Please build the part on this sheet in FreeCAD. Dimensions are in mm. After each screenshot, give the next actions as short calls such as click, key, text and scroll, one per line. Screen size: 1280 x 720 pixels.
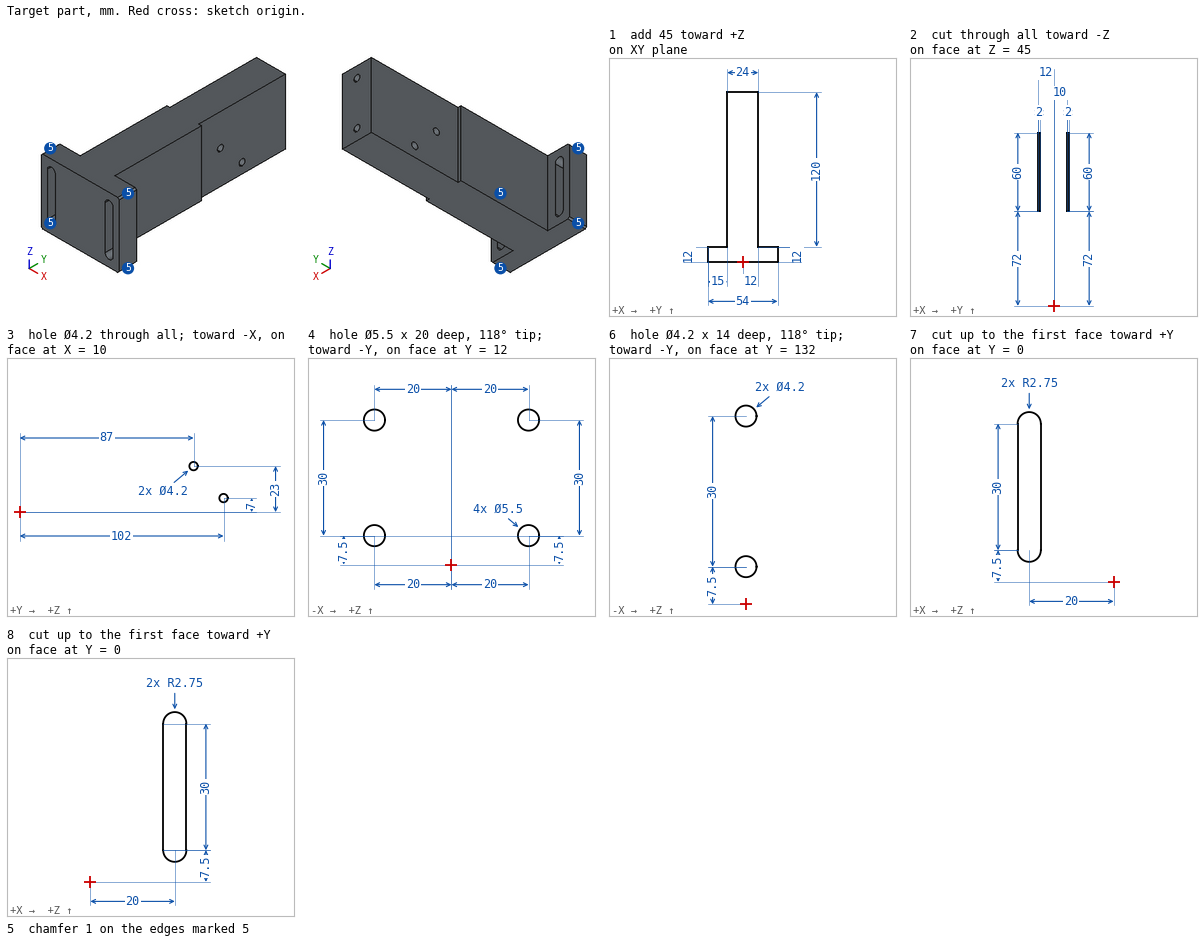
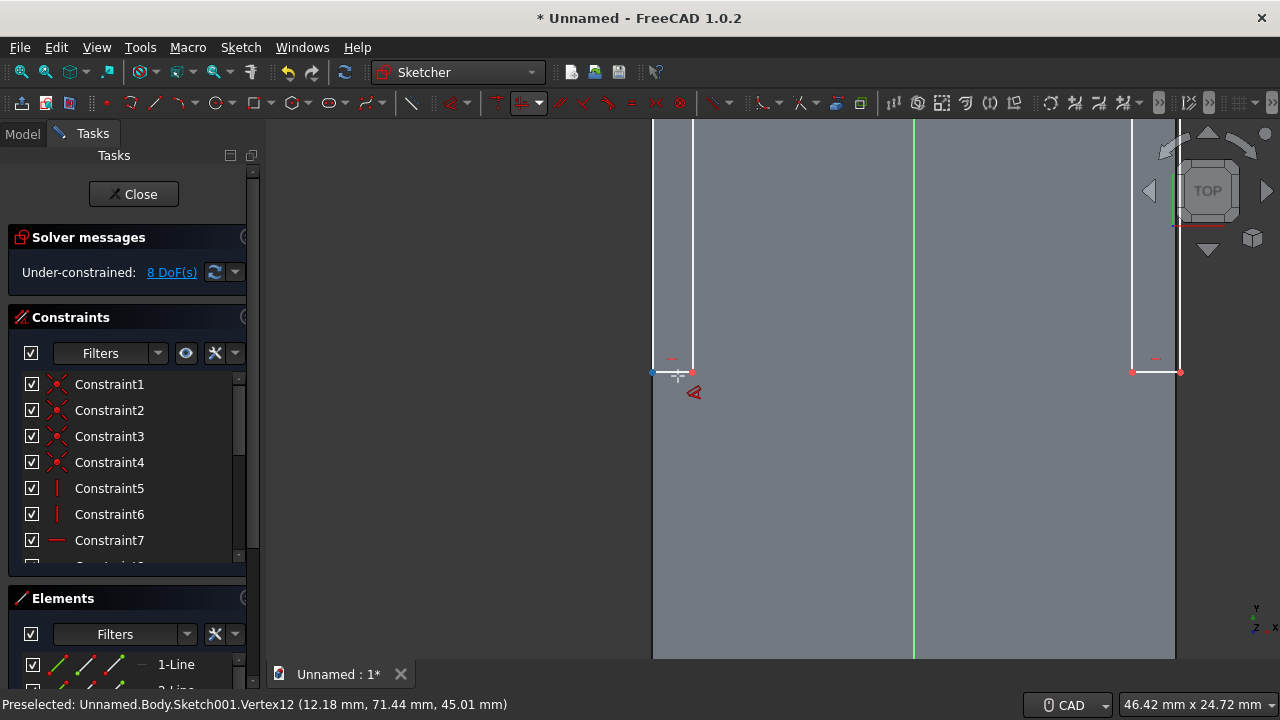
click(673, 372)
click(673, 338)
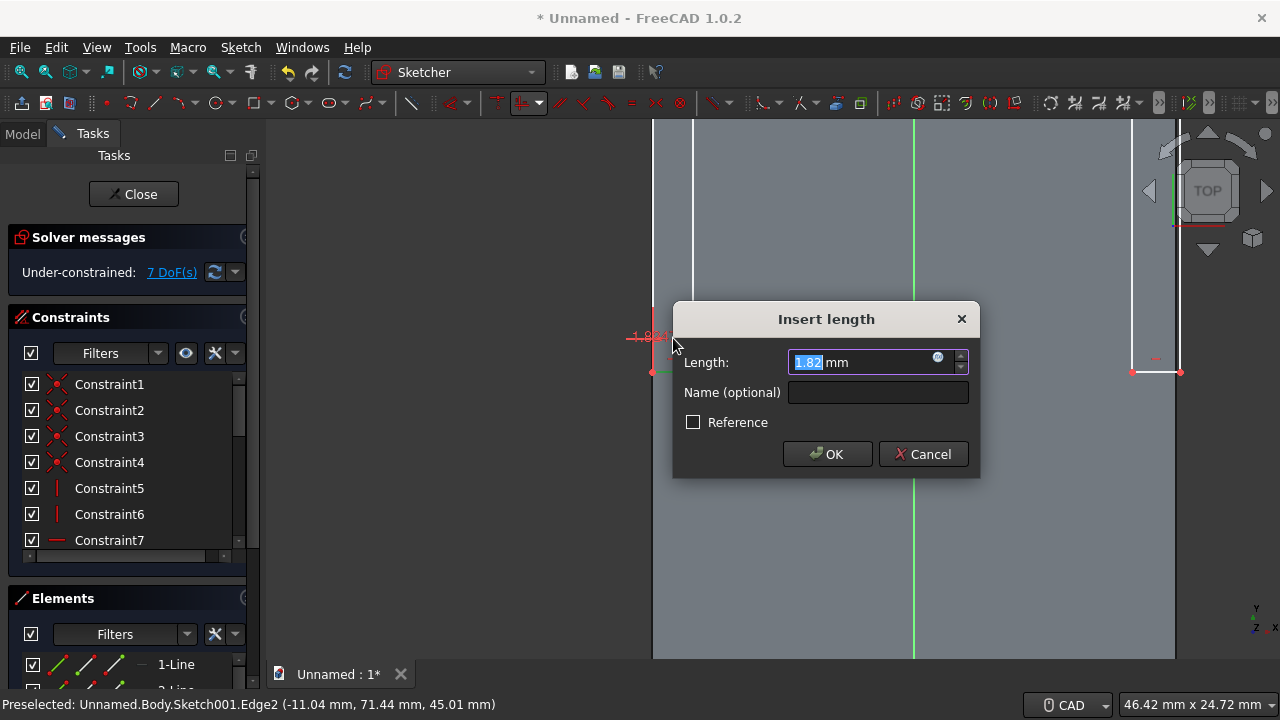
text(2)
key(Return)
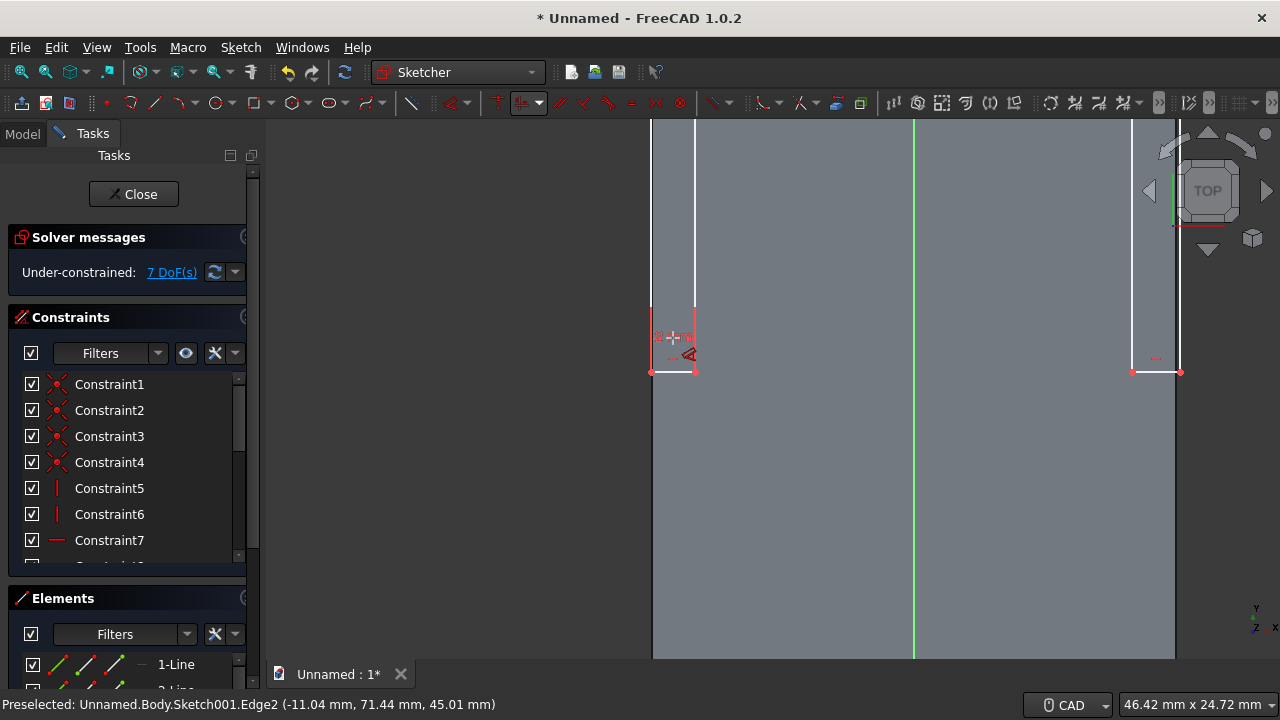
scroll(678, 376, down, 11)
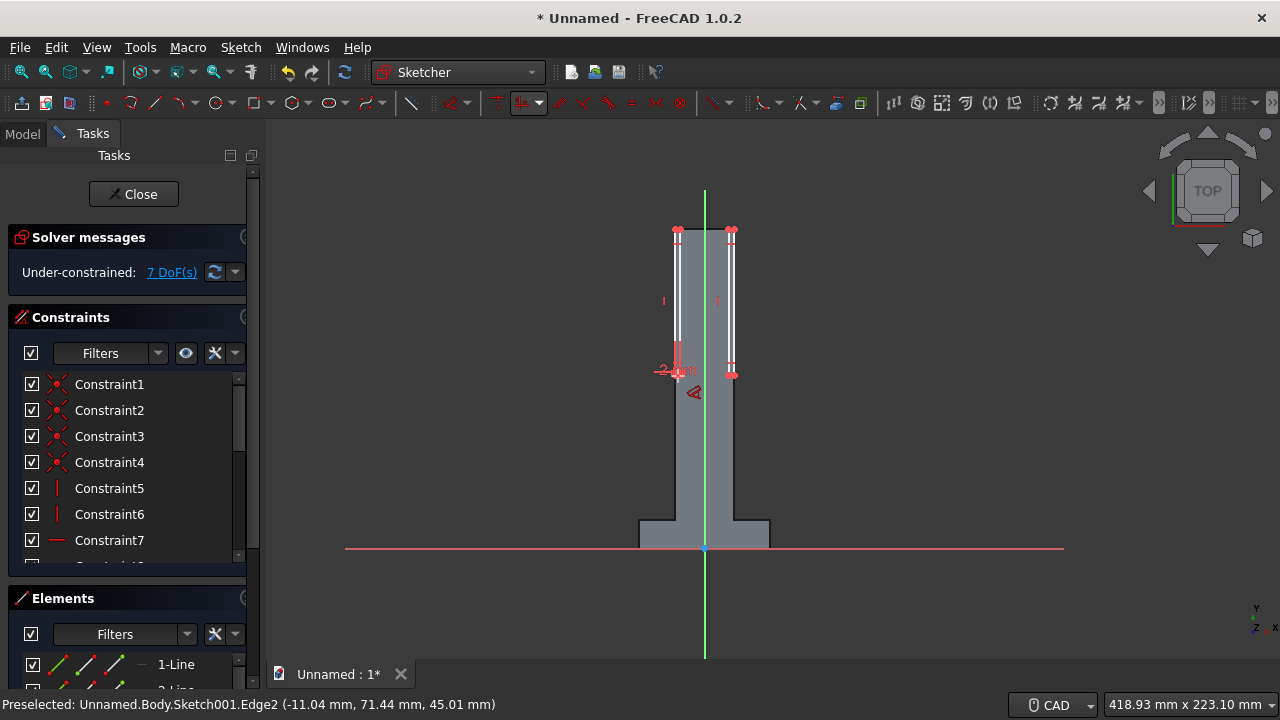
scroll(730, 376, up, 11)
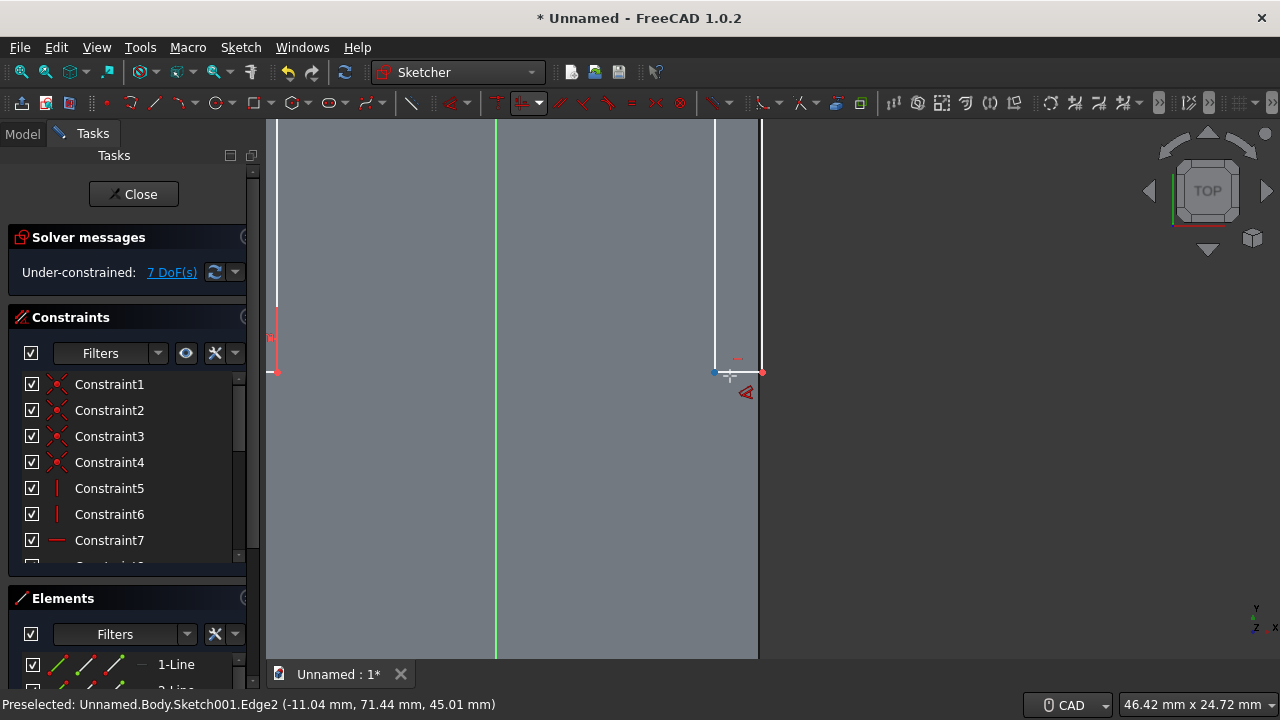
click(729, 372)
click(739, 338)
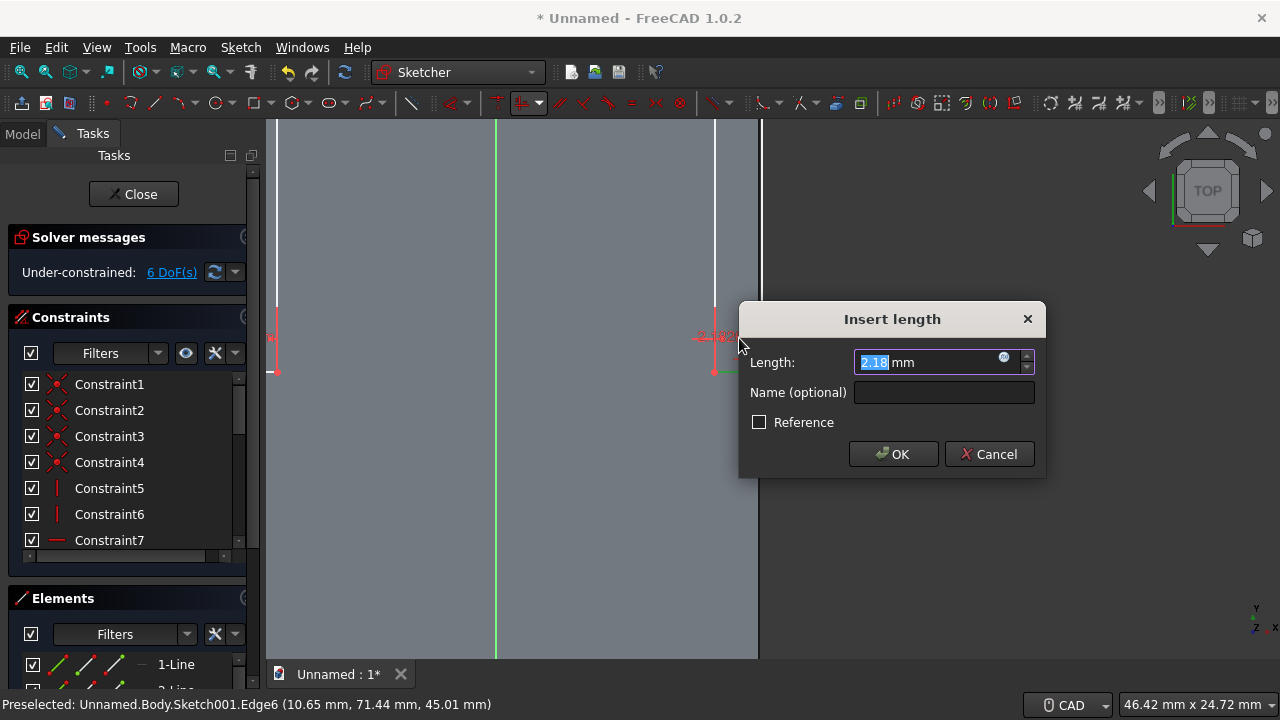
text(2)
key(Return)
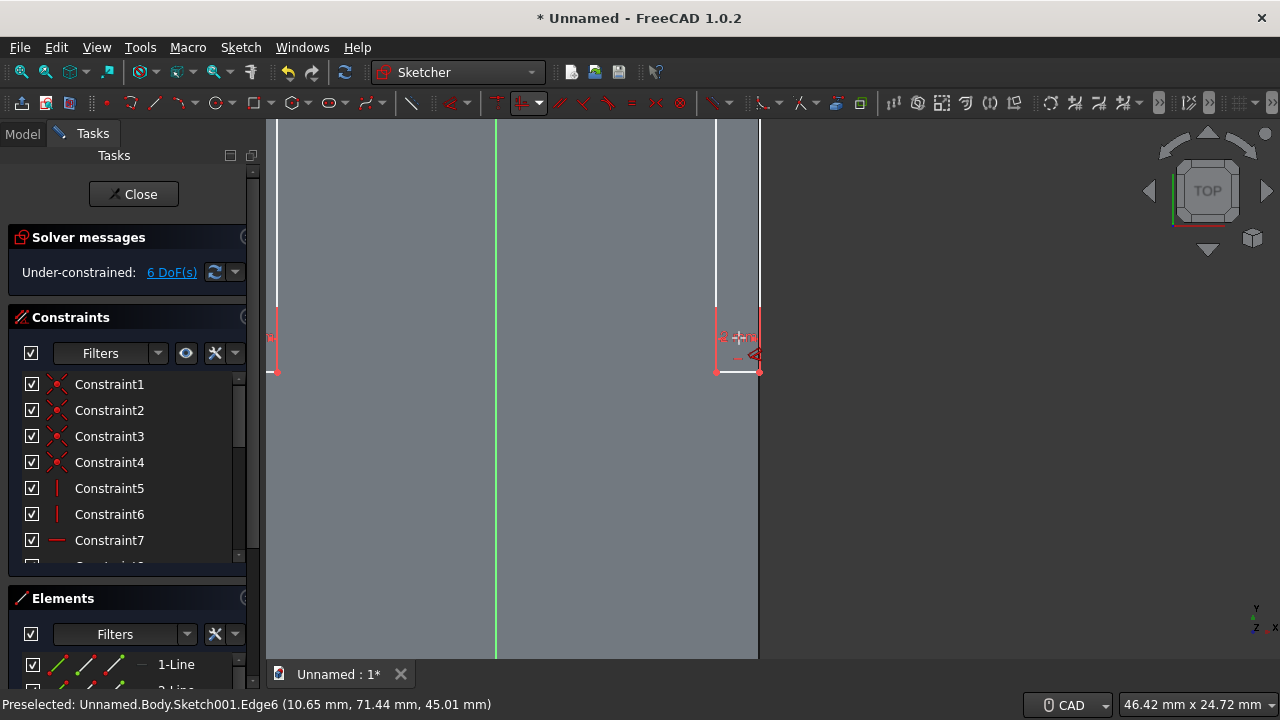
scroll(730, 376, down, 11)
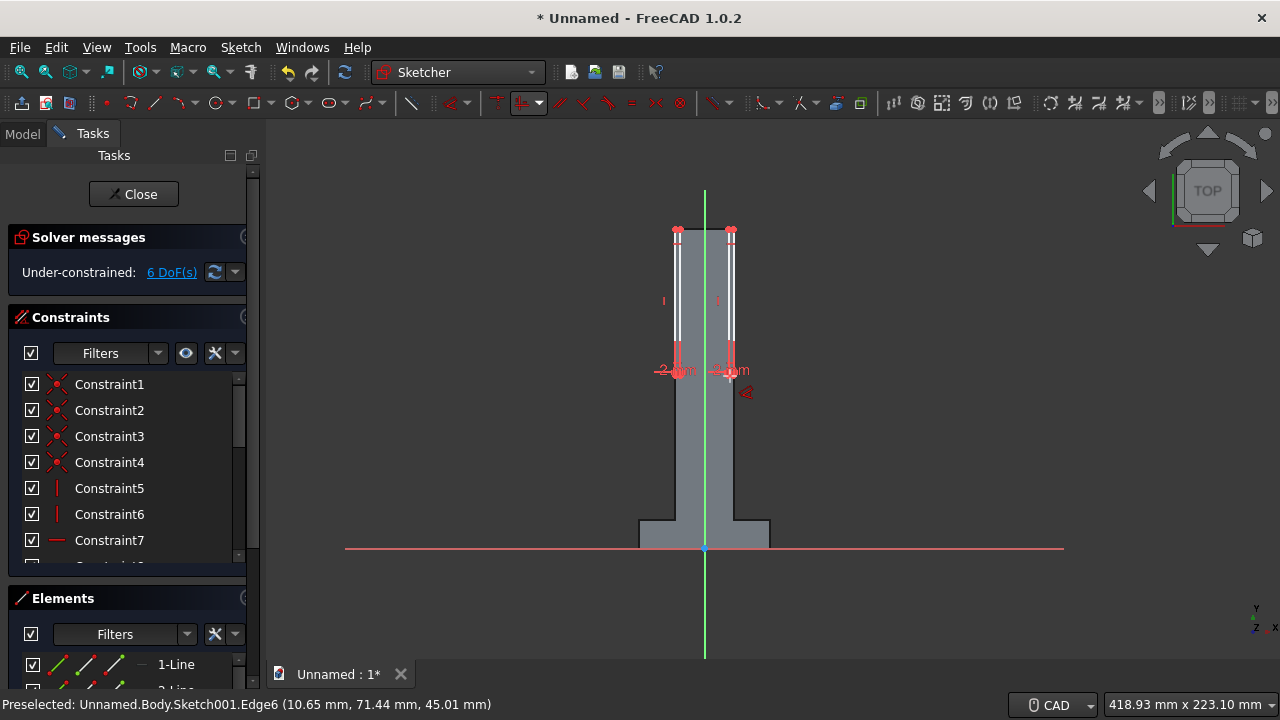
scroll(675, 274, up, 6)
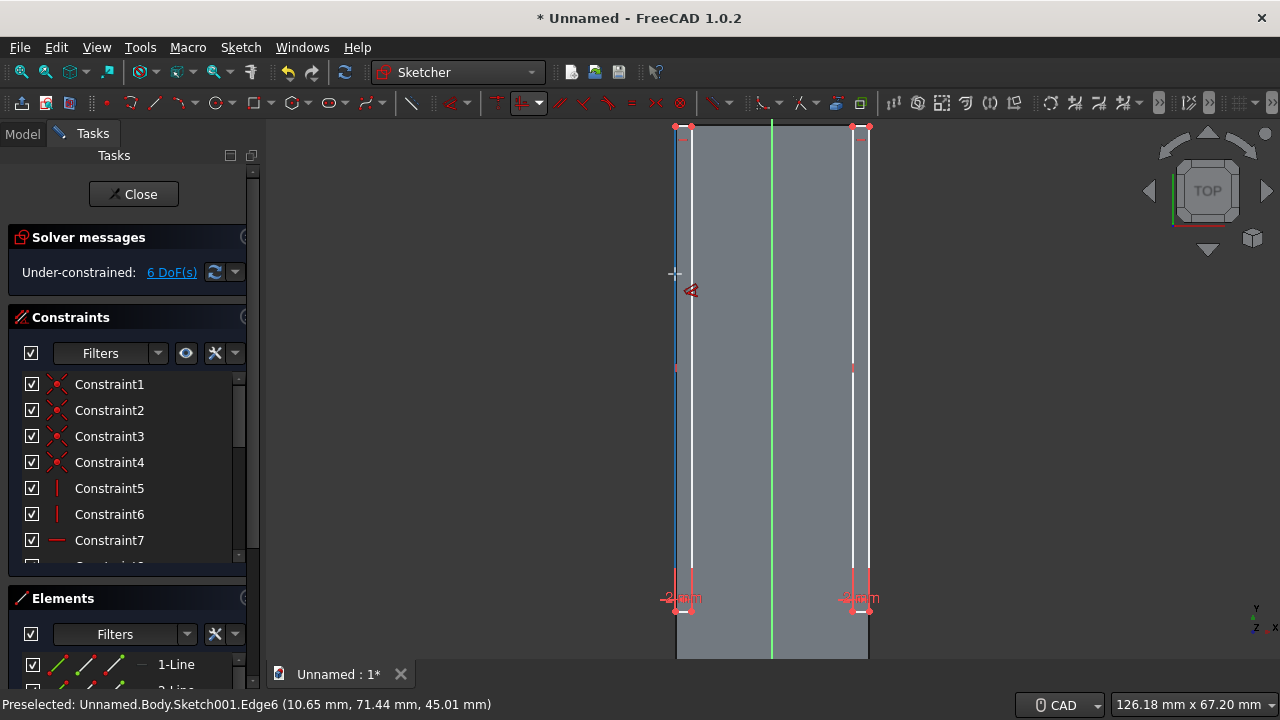
click(675, 272)
click(641, 379)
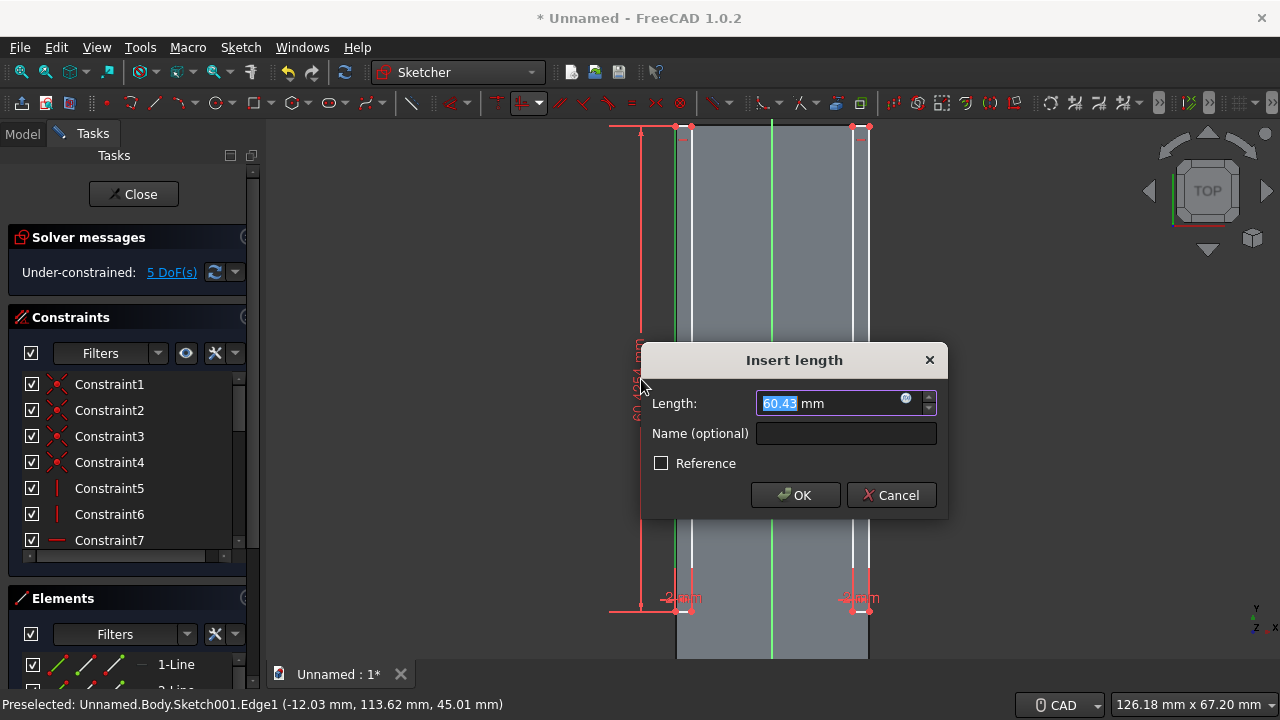
text(60)
key(Return)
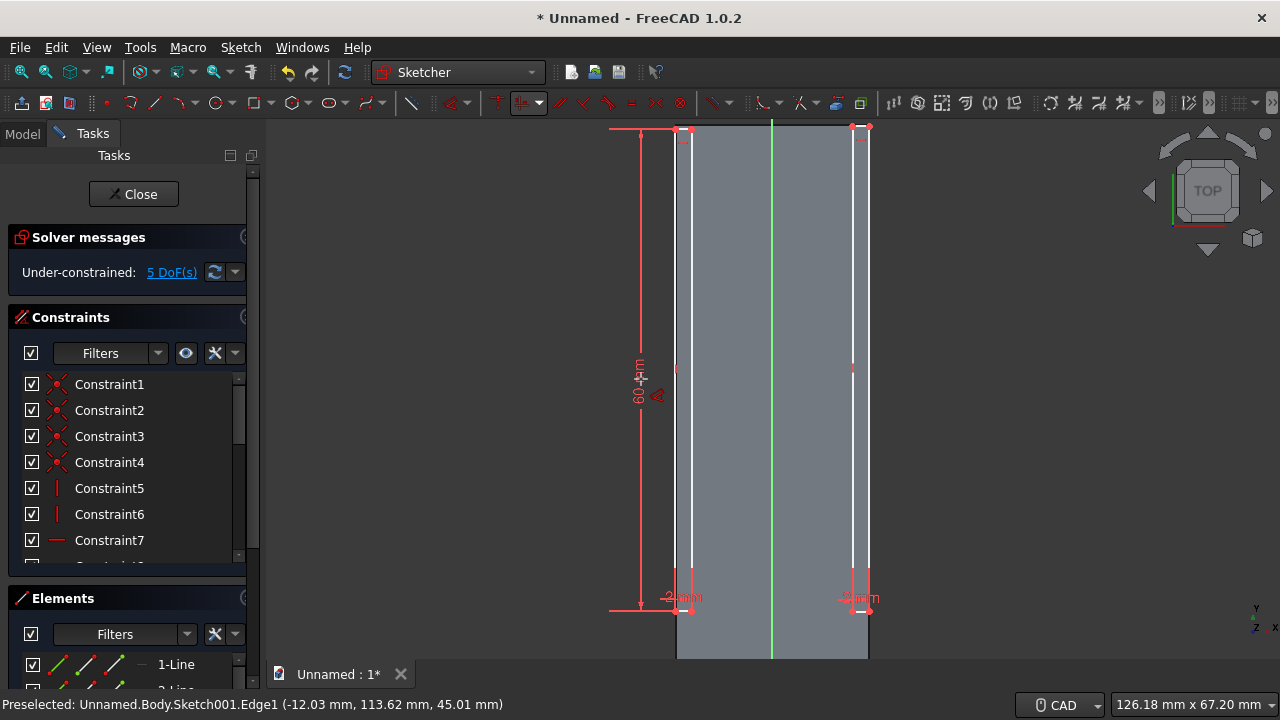
click(853, 272)
click(887, 379)